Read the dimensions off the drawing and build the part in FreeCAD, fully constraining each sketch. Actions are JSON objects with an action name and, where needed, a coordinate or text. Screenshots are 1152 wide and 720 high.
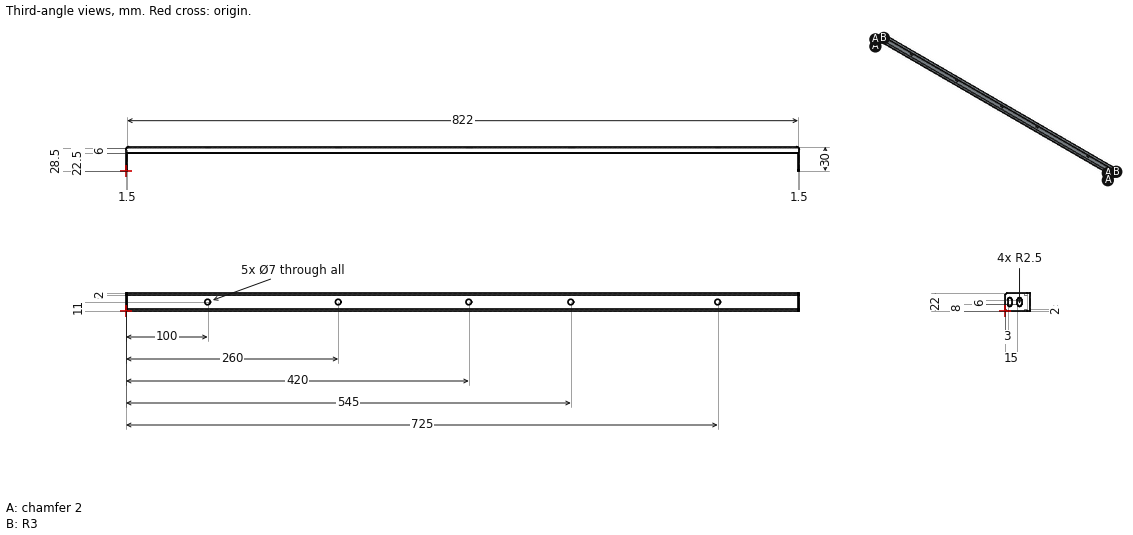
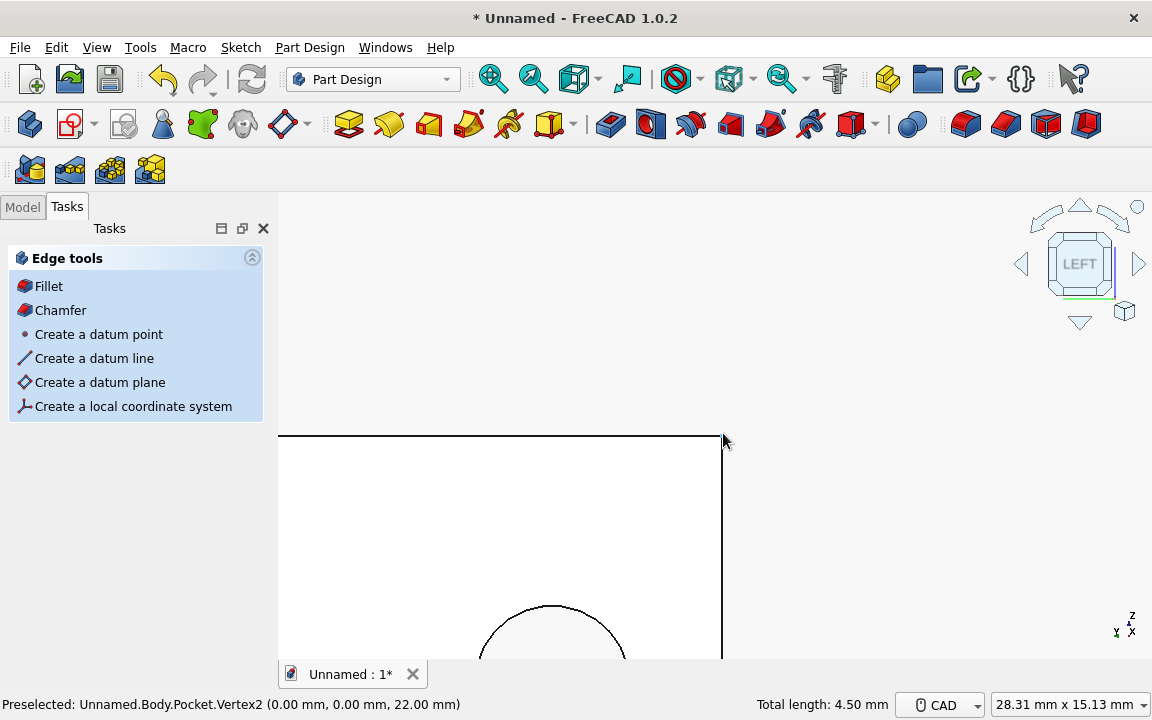
{"action": "left_click", "coordinate": [494, 80]}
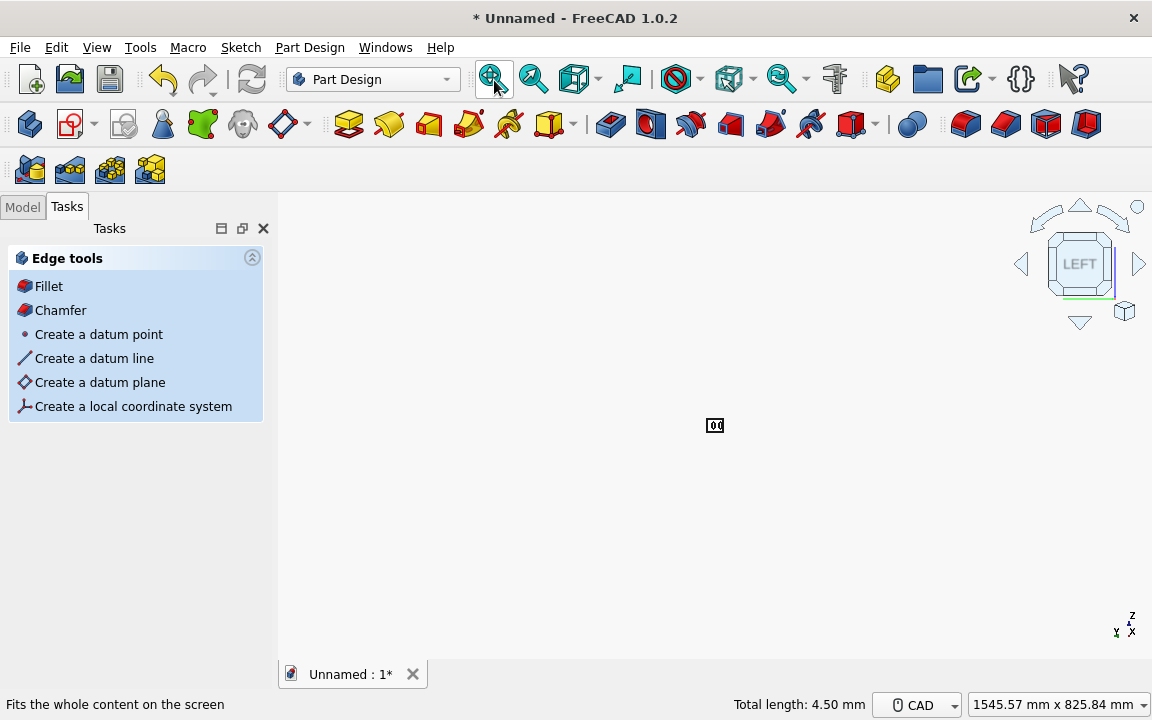
{"action": "key", "text": "v 3"}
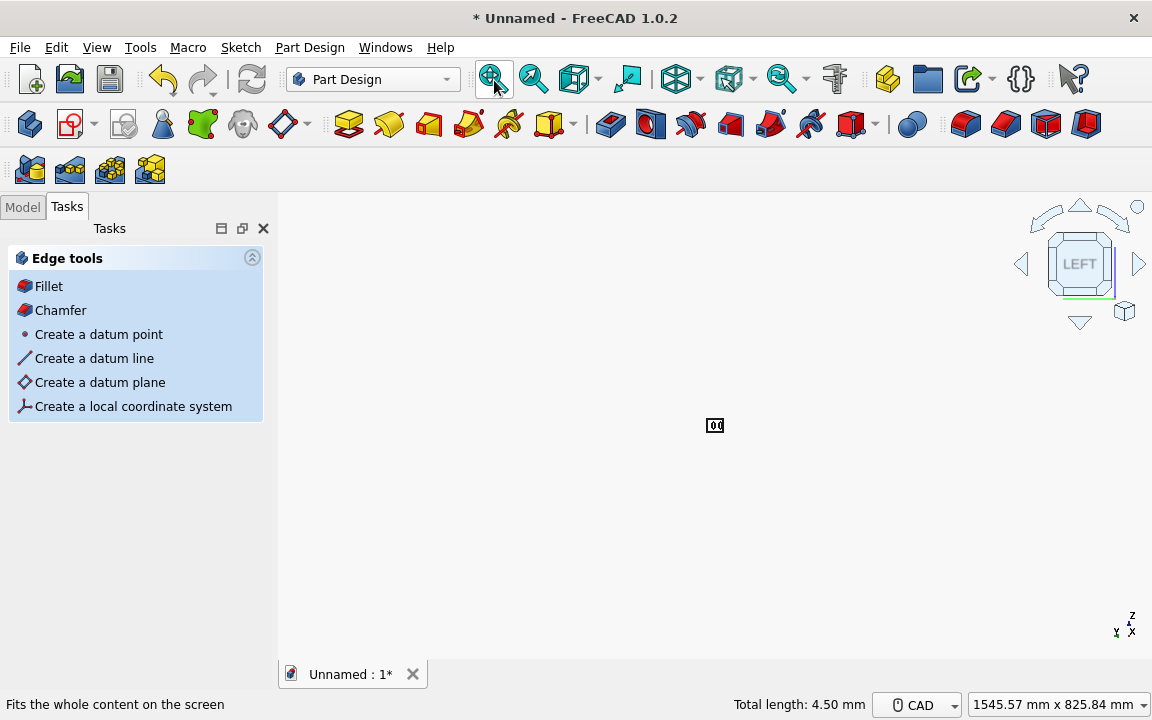
{"action": "key", "text": "0"}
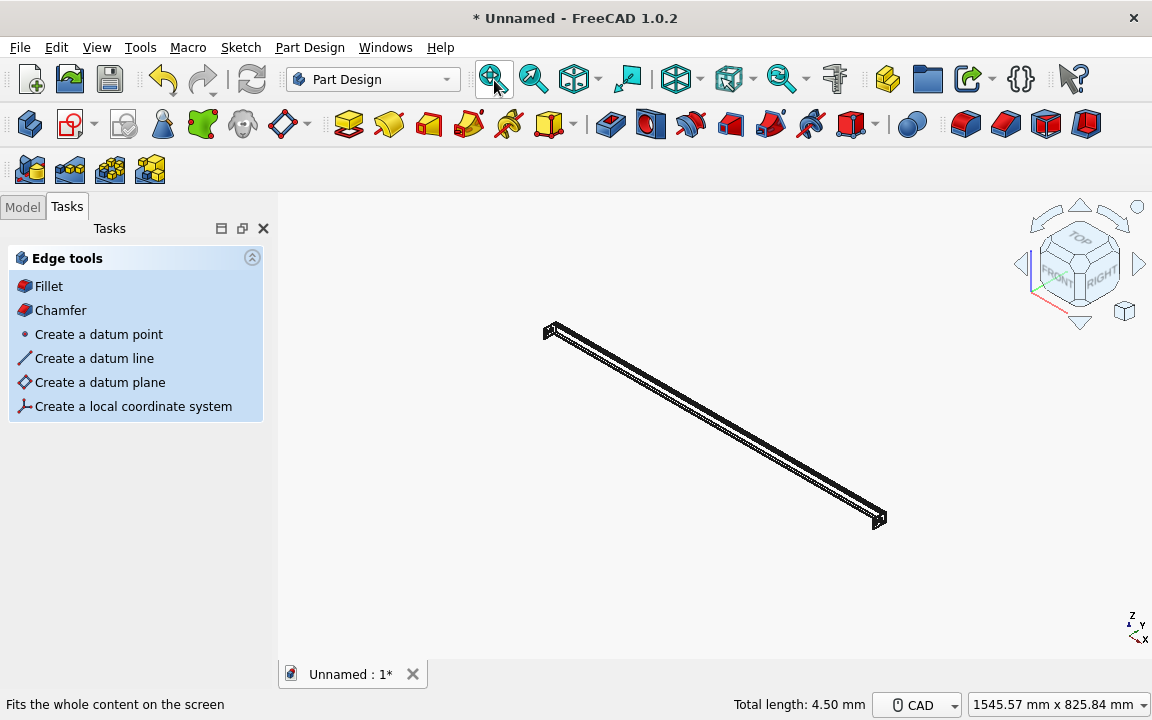
{"action": "left_click", "coordinate": [494, 80]}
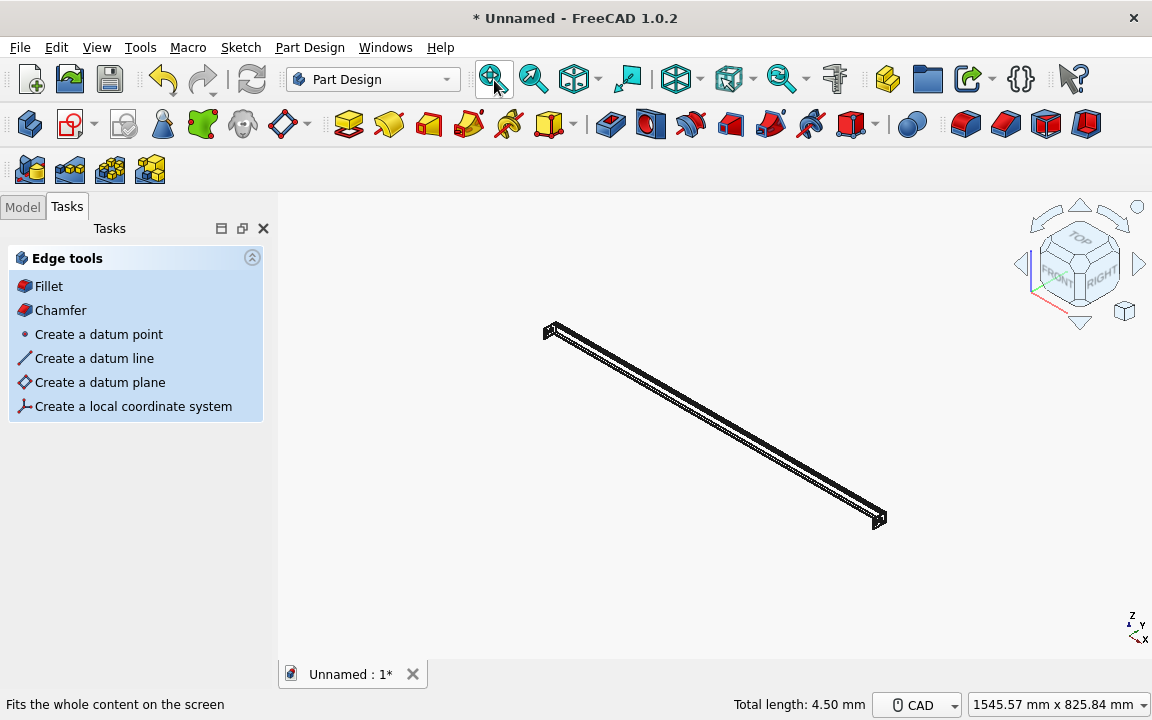
{"action": "scroll", "coordinate": [874, 518], "scroll_direction": "up", "scroll_amount": 15}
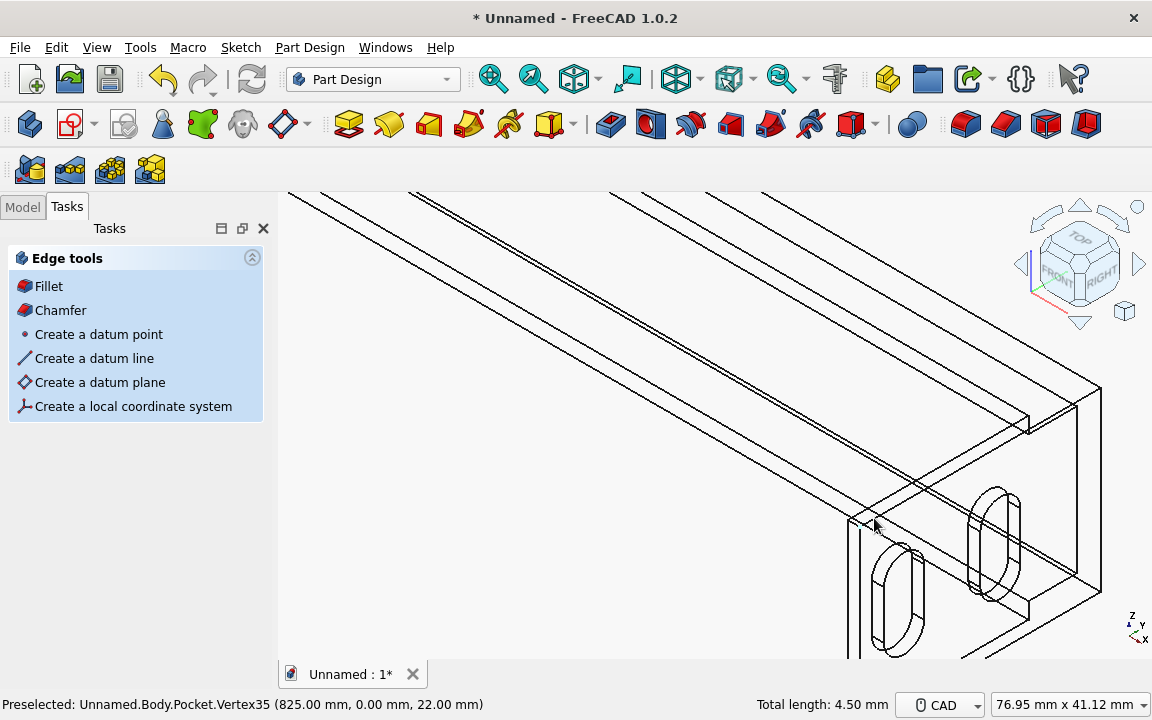
{"action": "left_click", "coordinate": [854, 523], "text": "ctrl"}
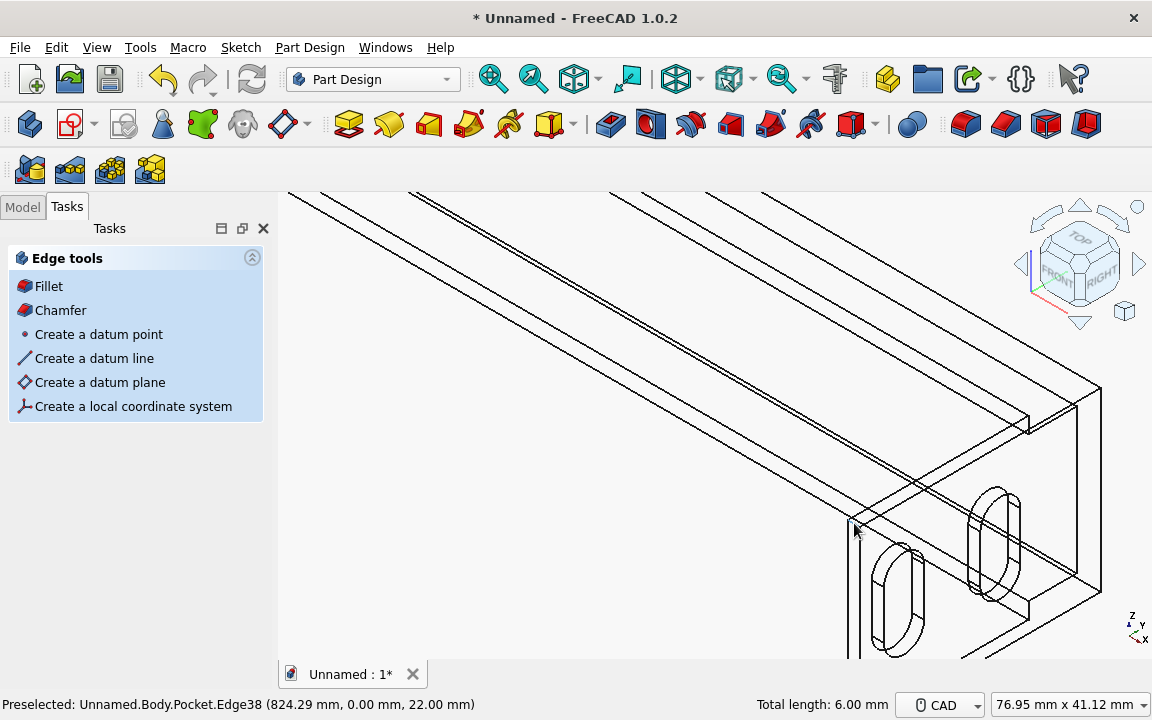
{"action": "key", "text": "v 1"}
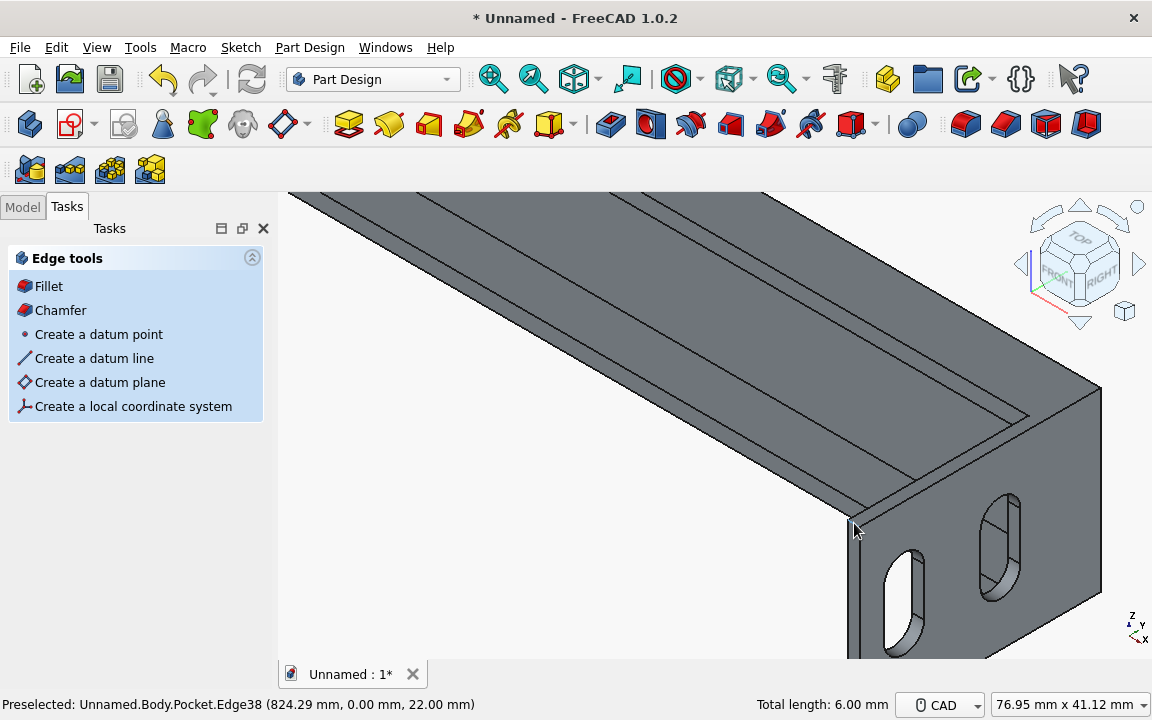
{"action": "left_click", "coordinate": [1006, 124]}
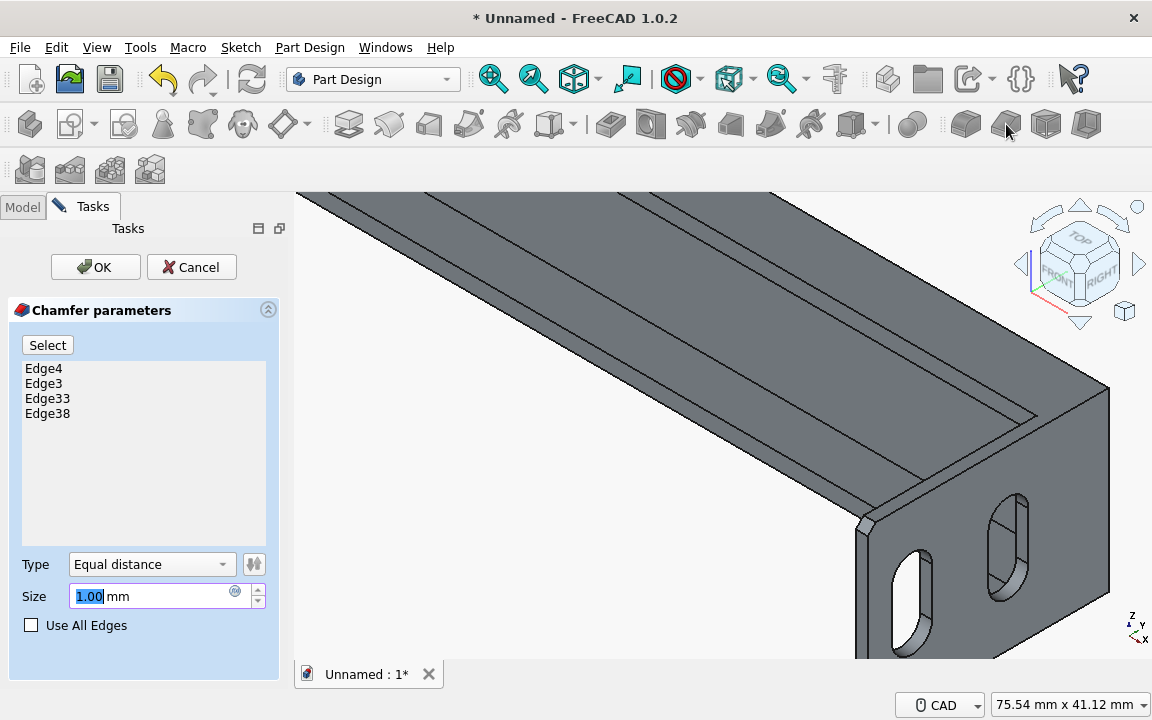
{"action": "type", "text": "2"}
{"action": "key", "text": "Tab"}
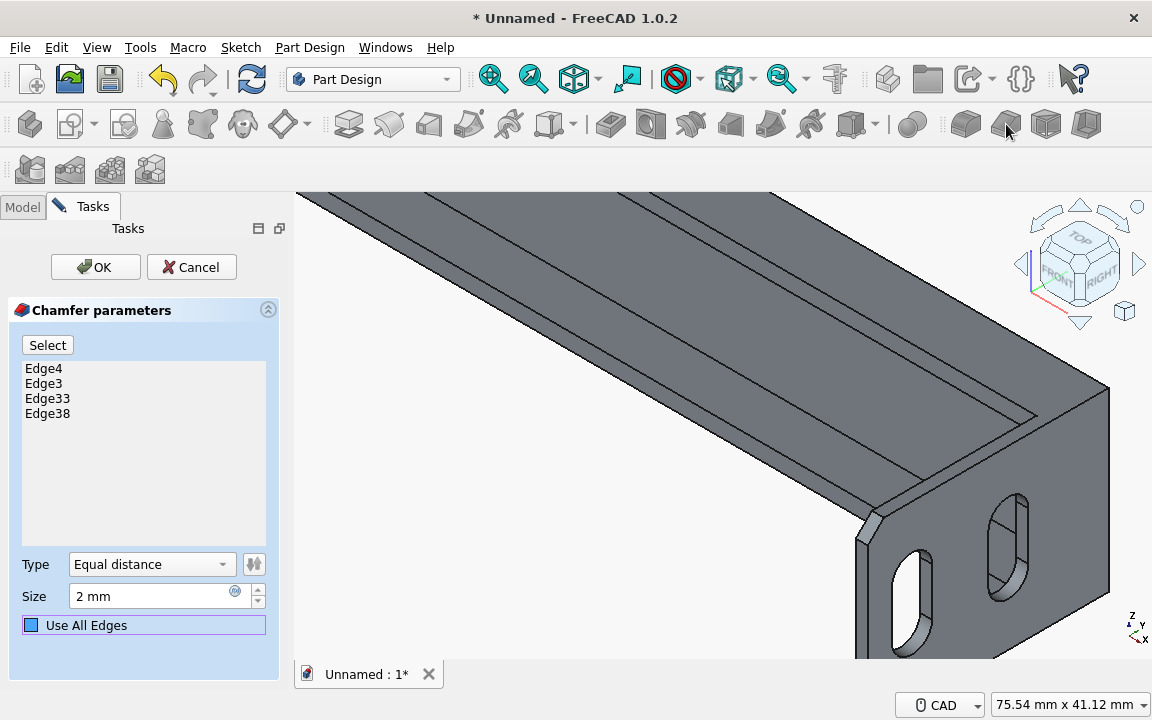
{"action": "left_click", "coordinate": [96, 267]}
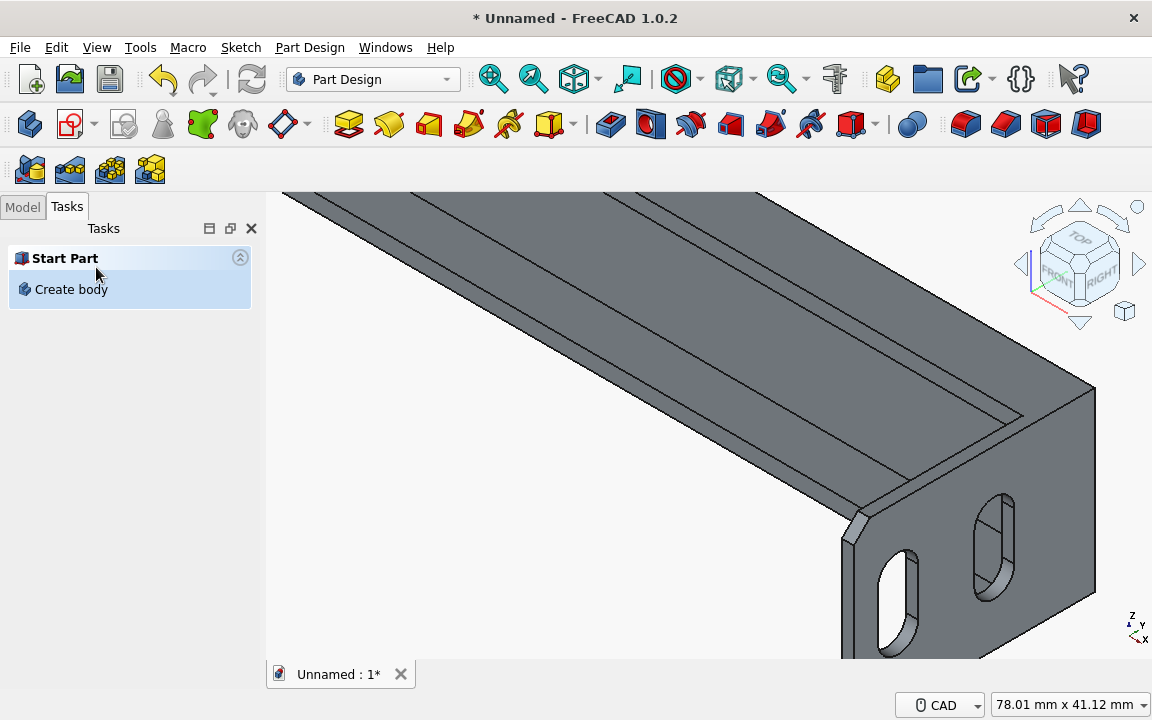
{"action": "left_click", "coordinate": [494, 80]}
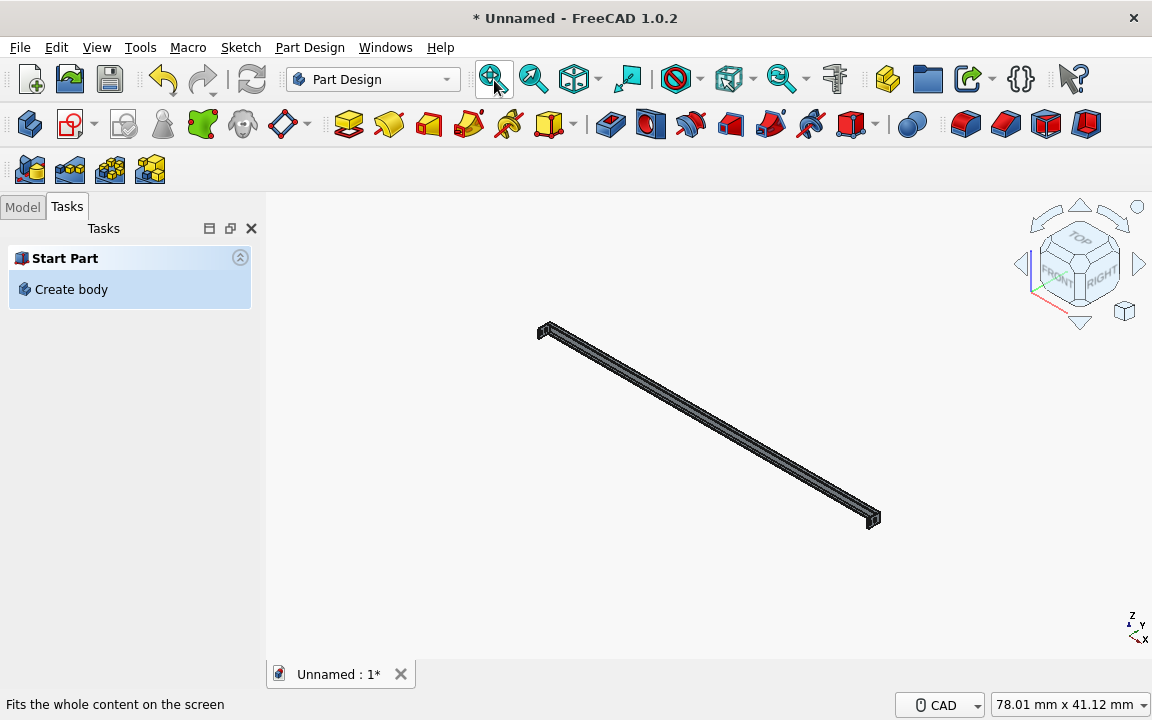
{"action": "scroll", "coordinate": [550, 326], "scroll_direction": "up", "scroll_amount": 6}